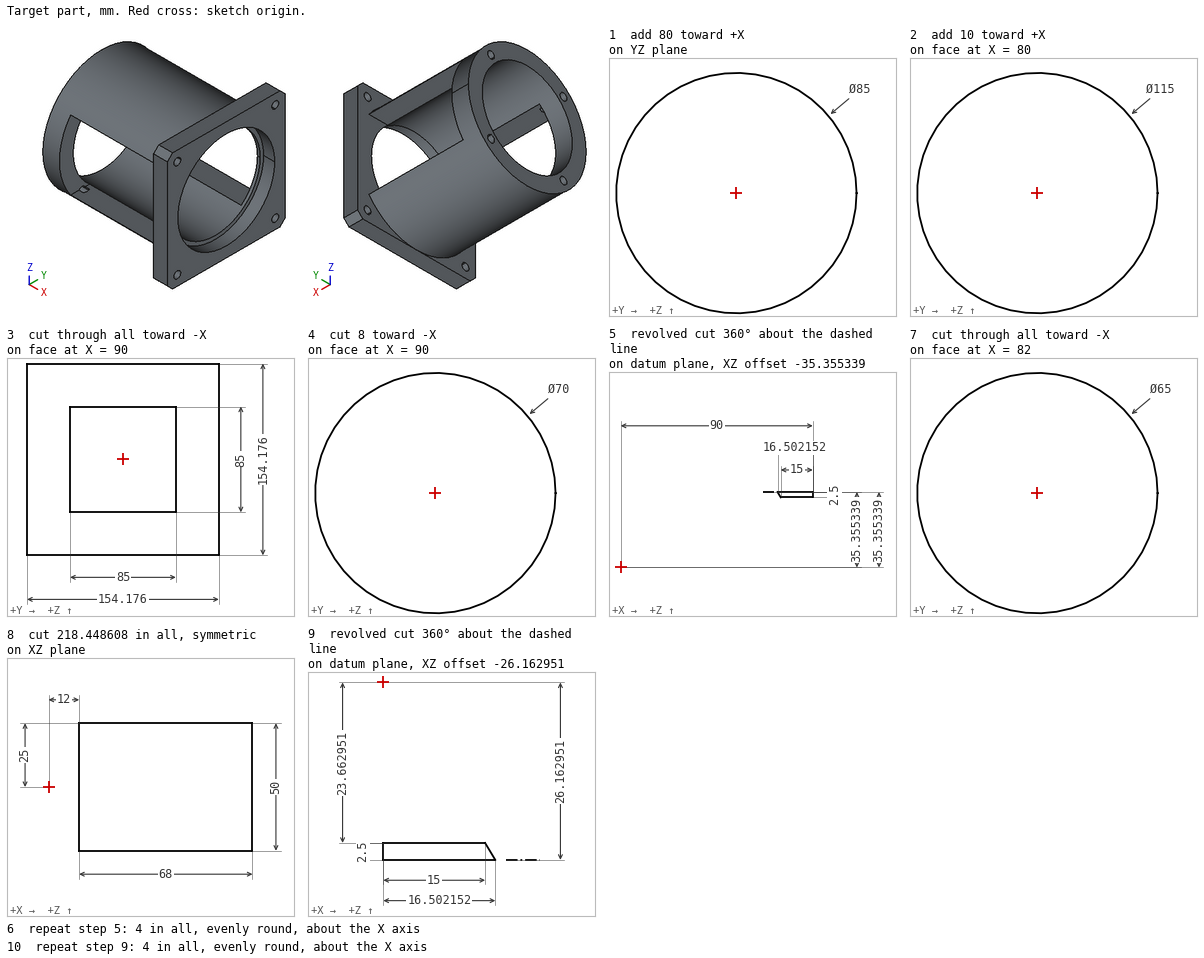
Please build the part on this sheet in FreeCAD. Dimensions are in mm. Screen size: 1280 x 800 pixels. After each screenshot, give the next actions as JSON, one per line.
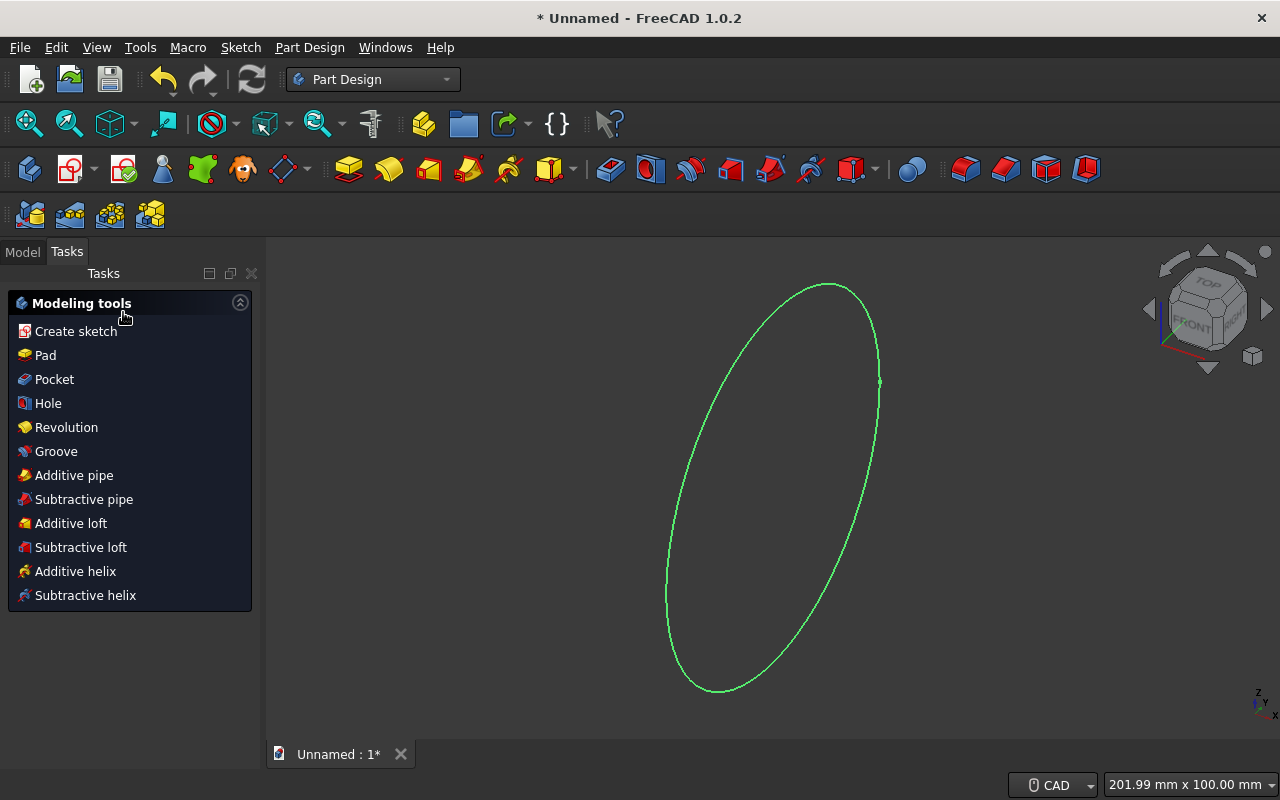
{"action": "left_click", "coordinate": [350, 170]}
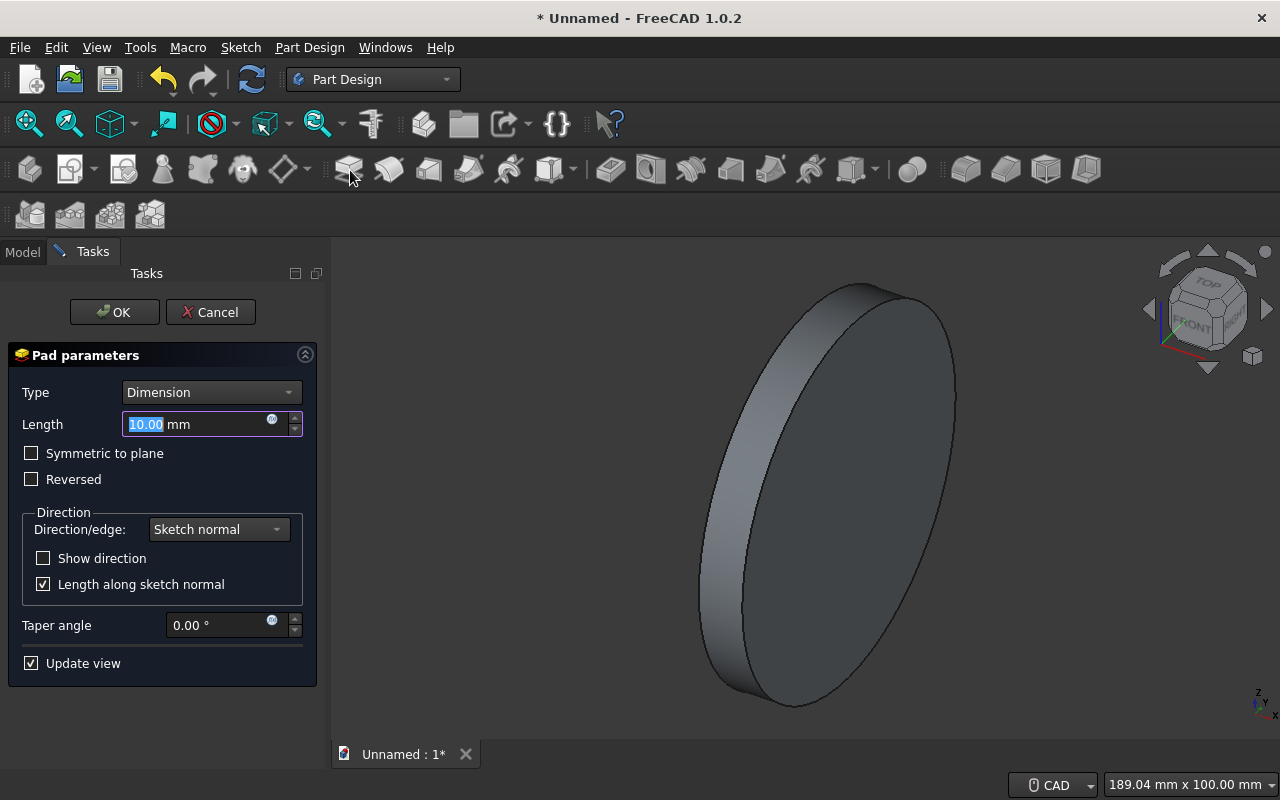
{"action": "type", "text": "80"}
{"action": "key", "text": "Tab"}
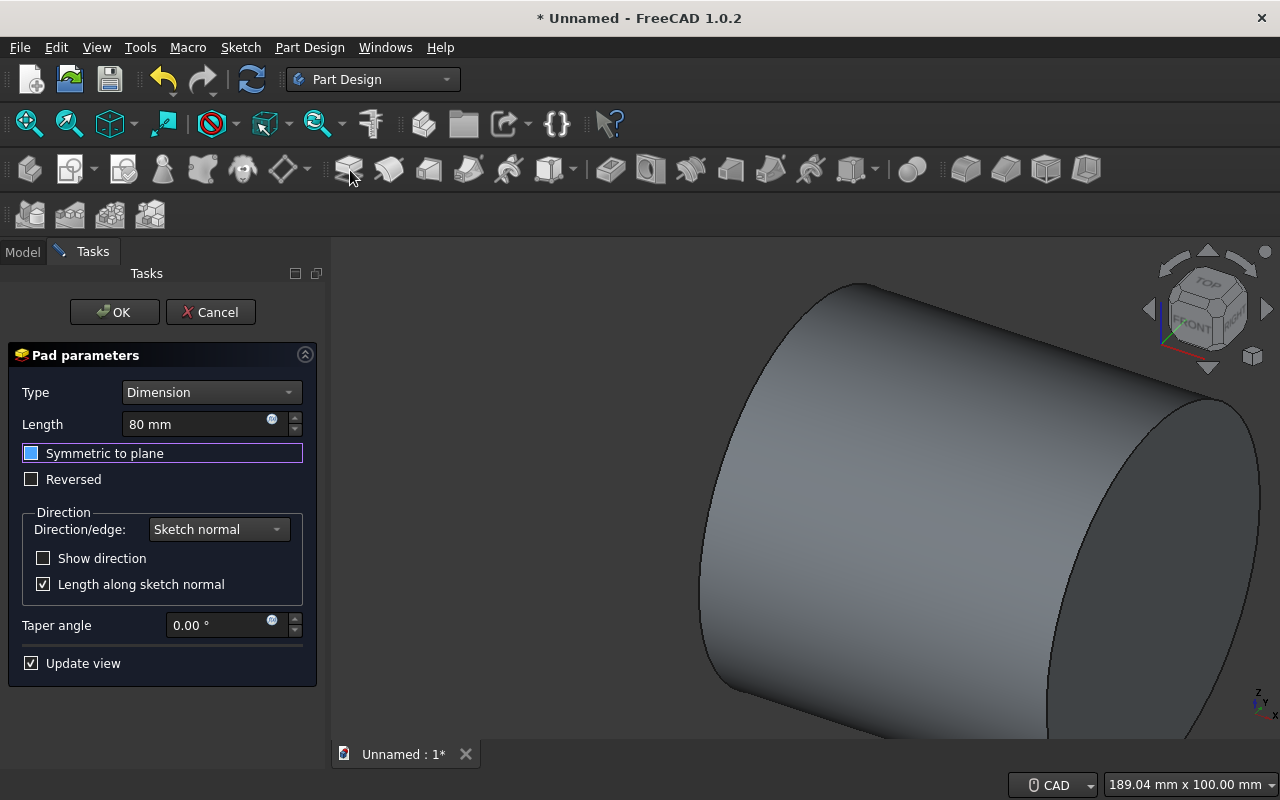
{"action": "left_click", "coordinate": [115, 312]}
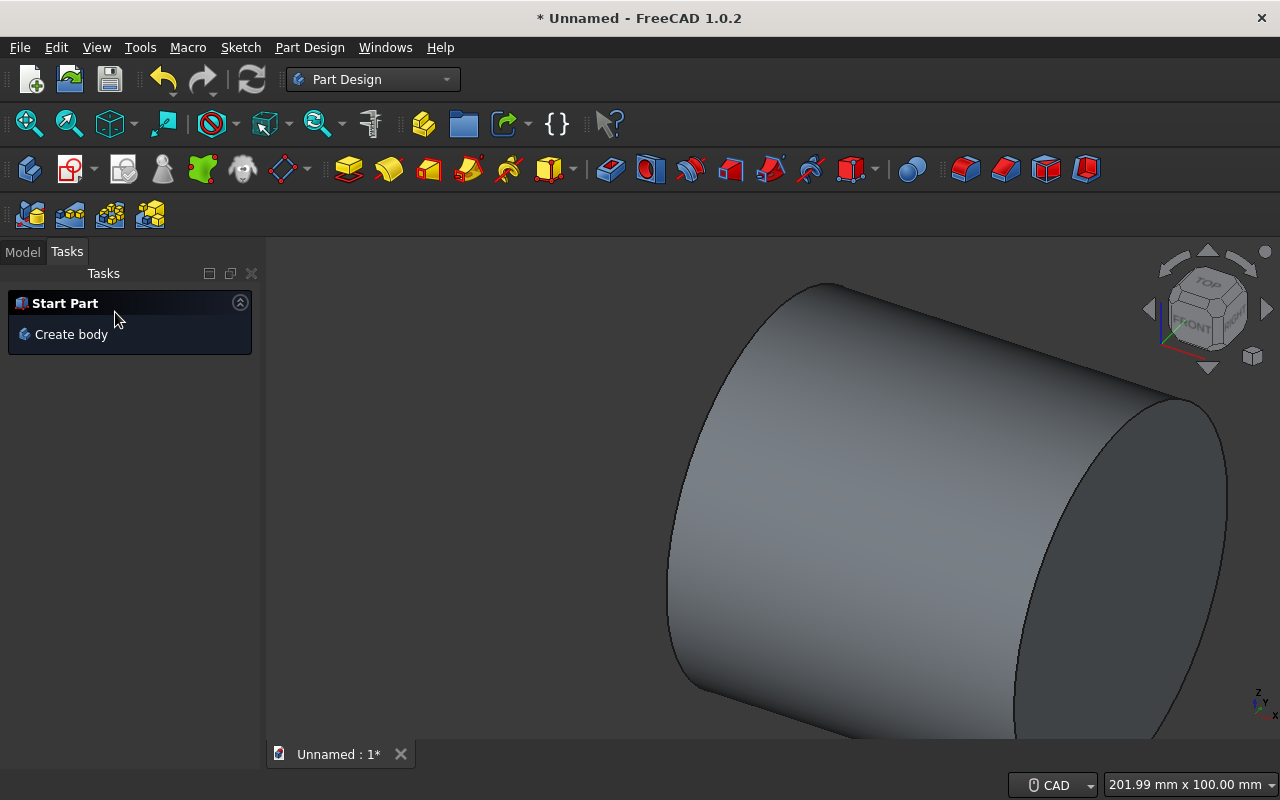
{"action": "left_click", "coordinate": [30, 124]}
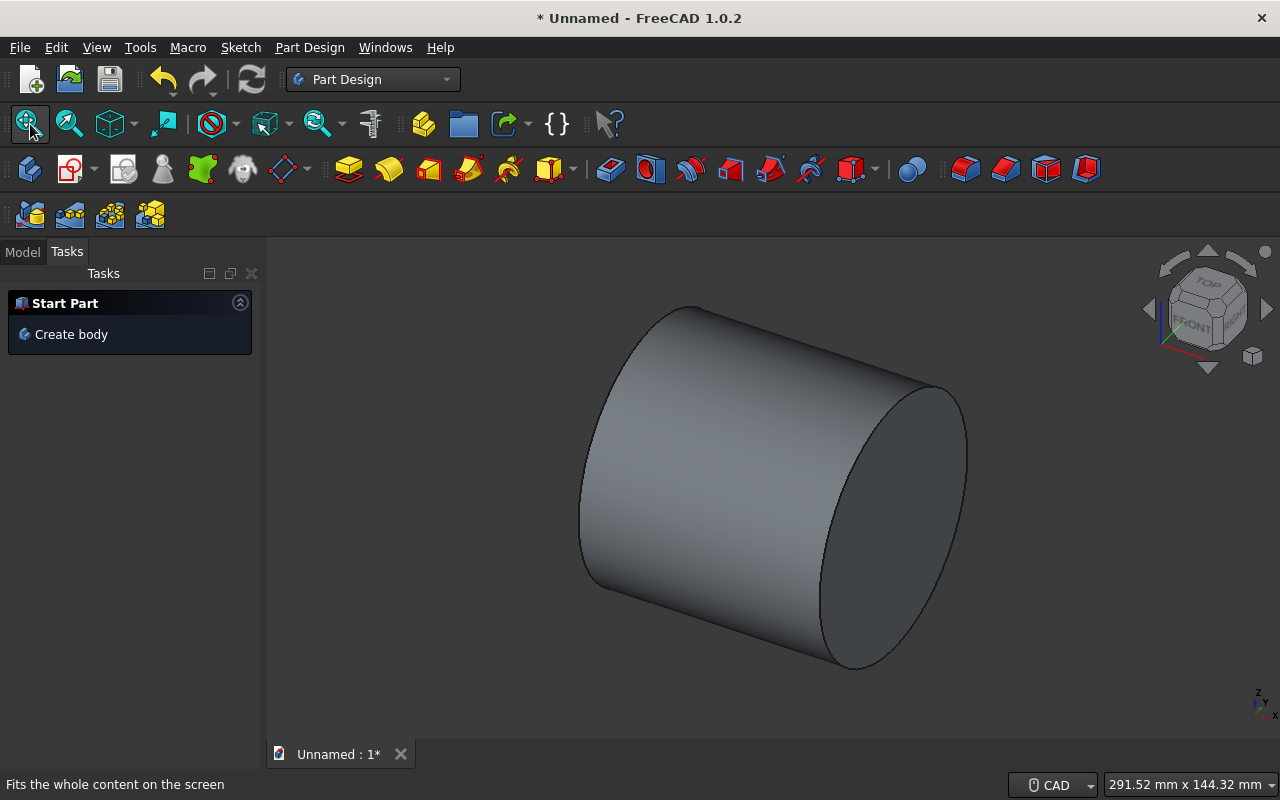
{"action": "left_click", "coordinate": [893, 527]}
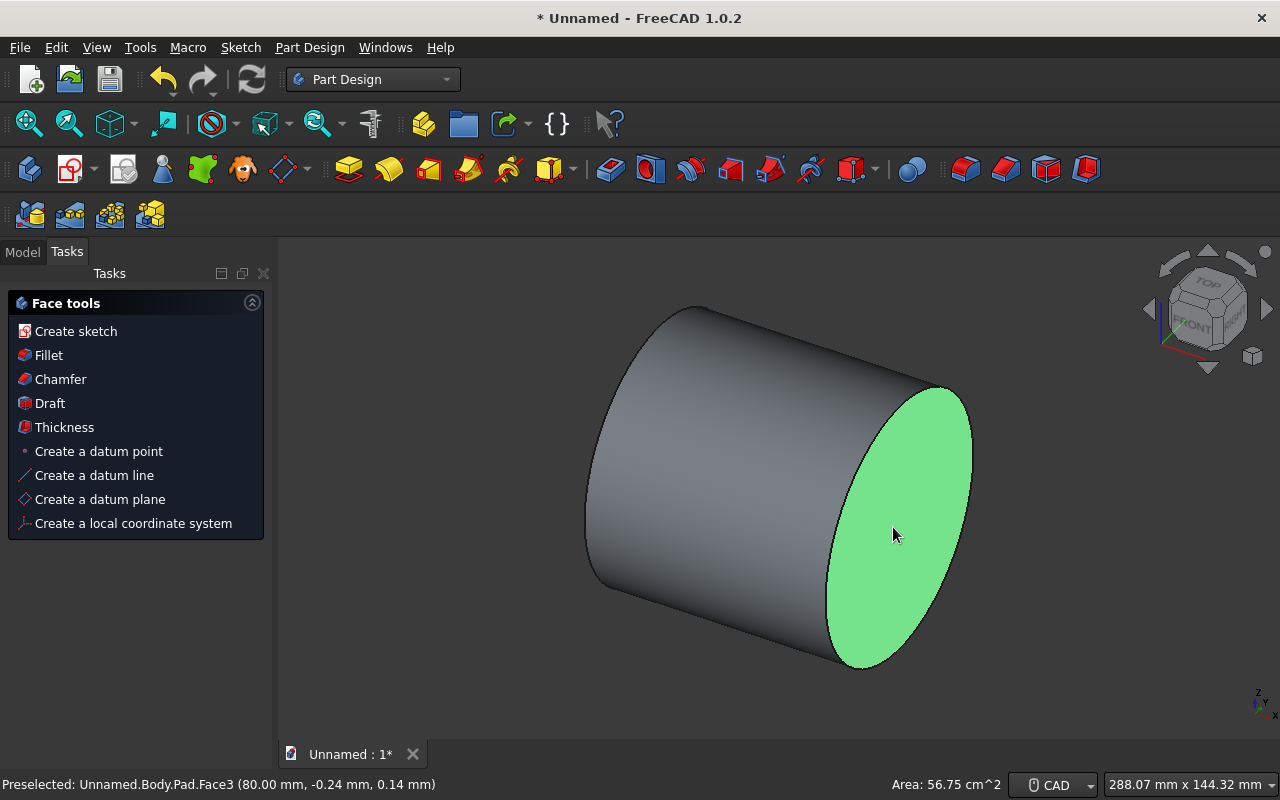
{"action": "left_click", "coordinate": [70, 170]}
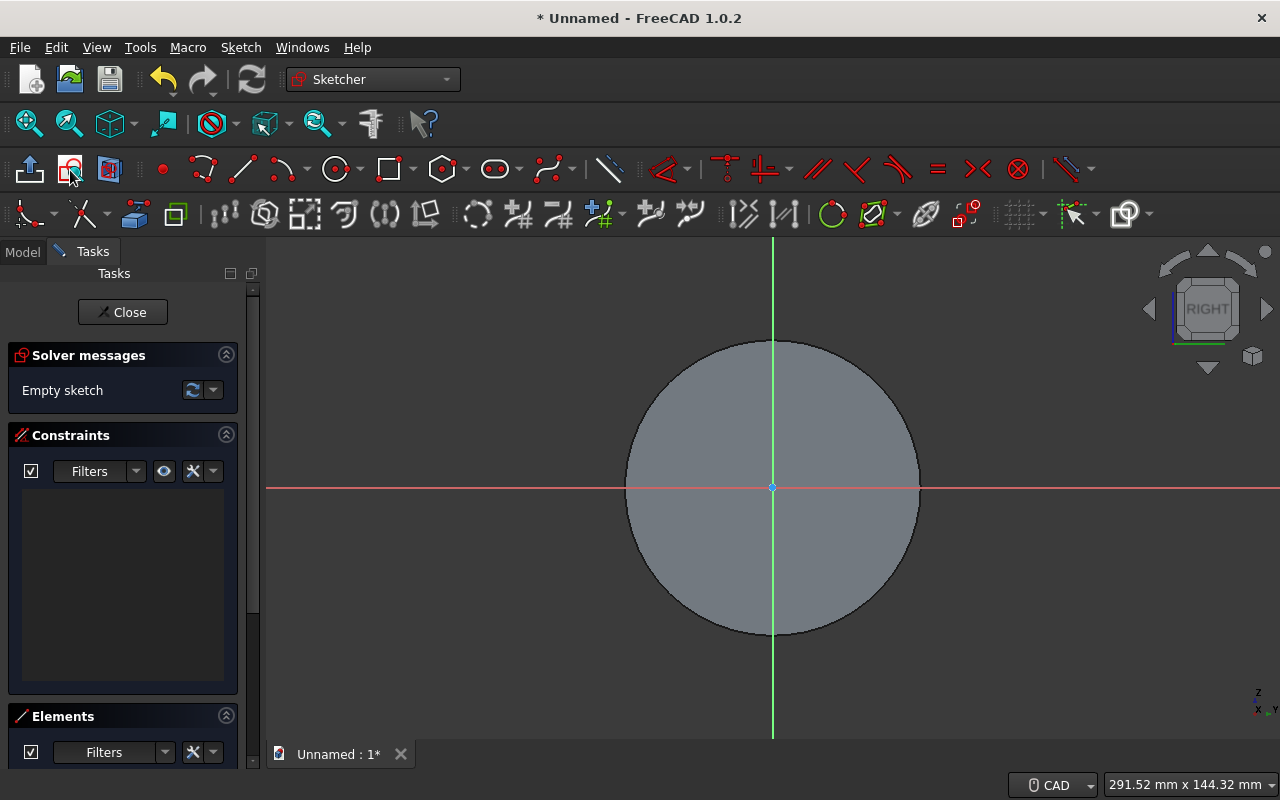
{"action": "scroll", "coordinate": [396, 488], "scroll_direction": "down", "scroll_amount": 1}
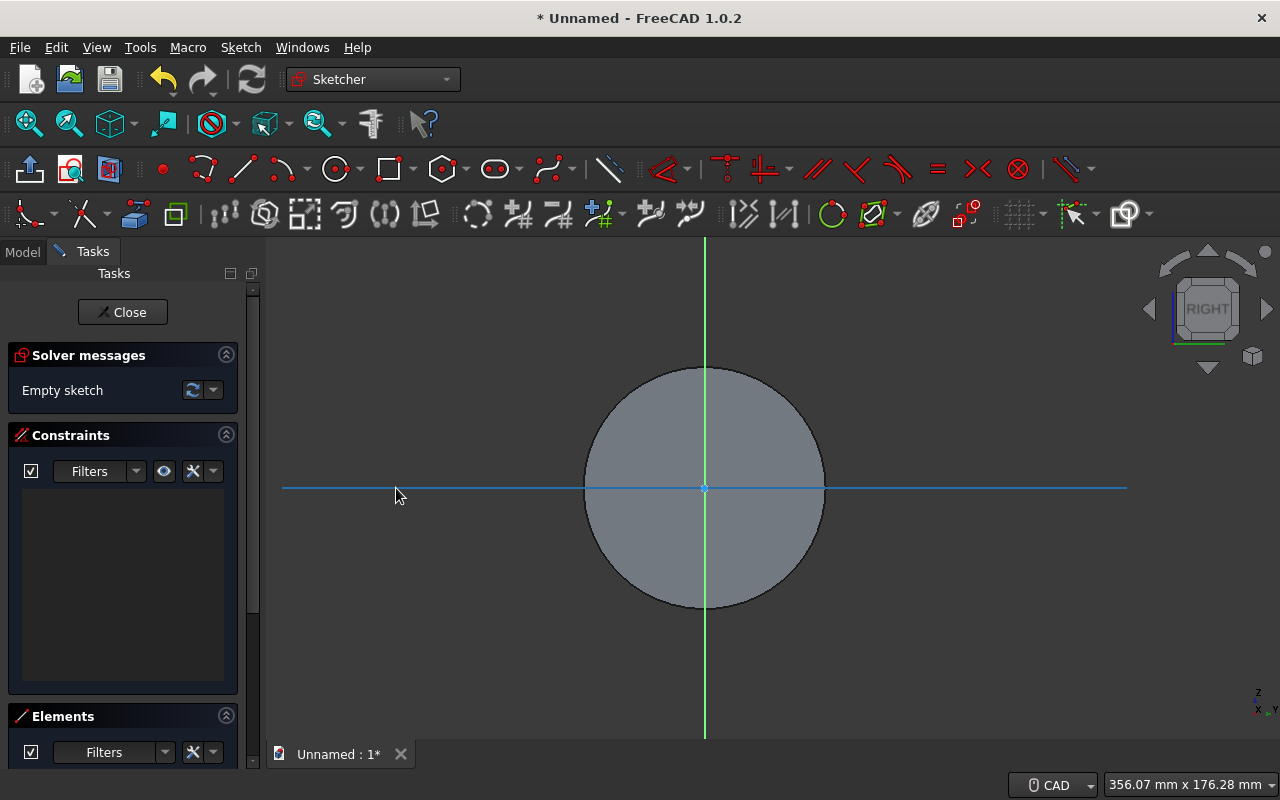
{"action": "left_click", "coordinate": [336, 170]}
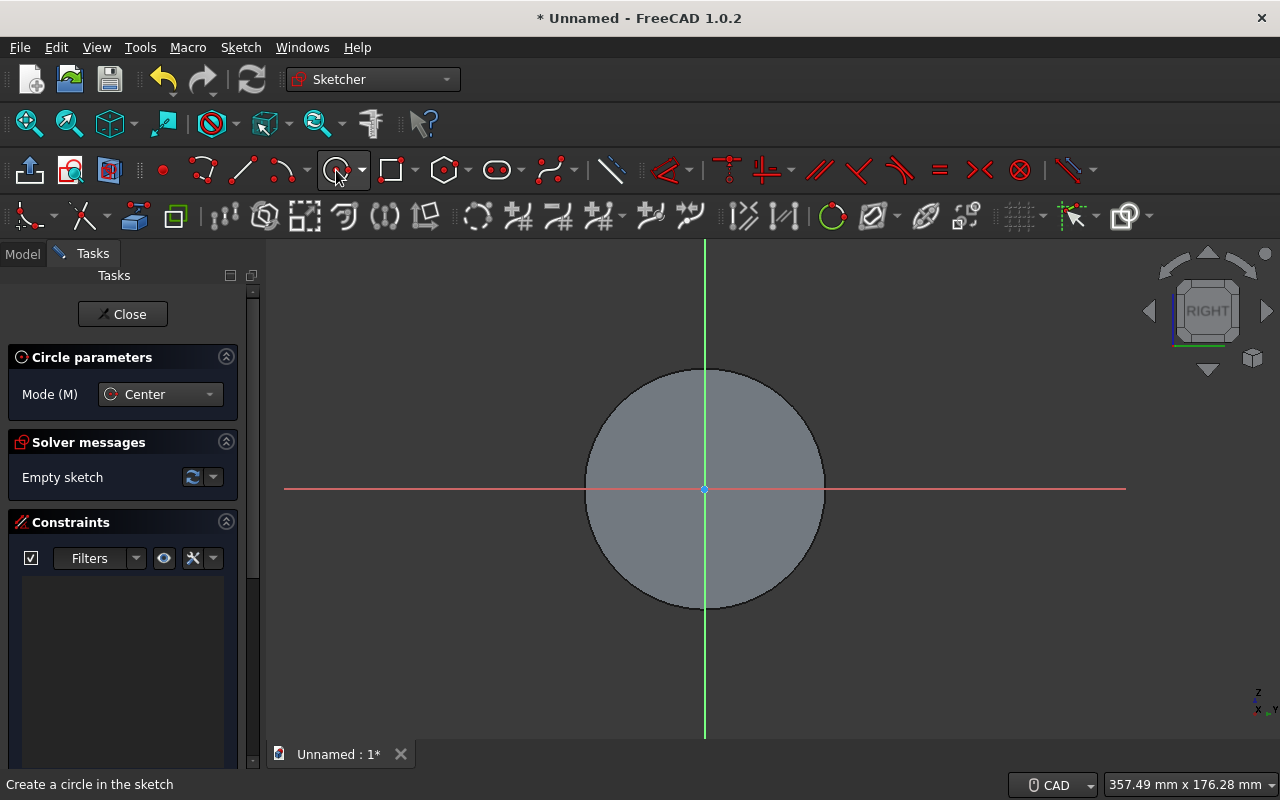
{"action": "left_click", "coordinate": [705, 489]}
{"action": "mouse_move", "coordinate": [820, 374]}